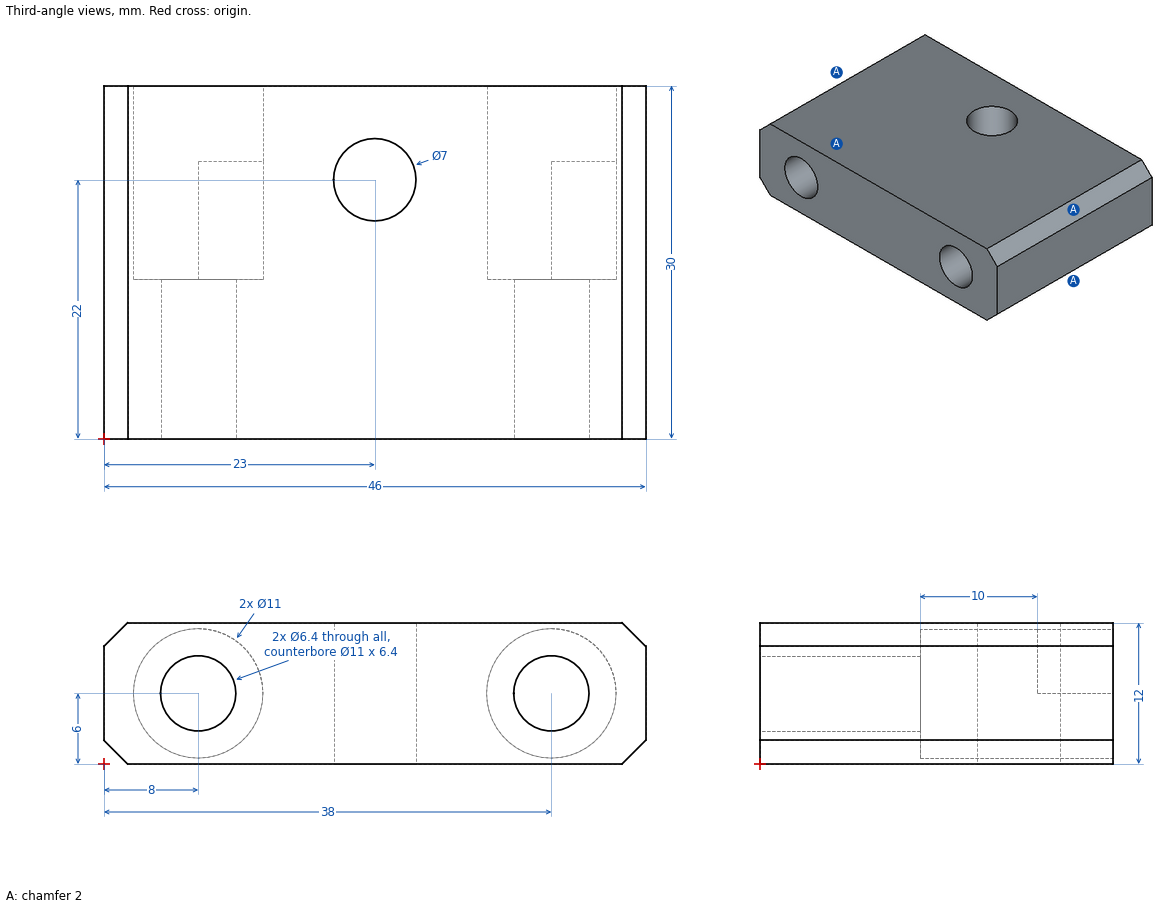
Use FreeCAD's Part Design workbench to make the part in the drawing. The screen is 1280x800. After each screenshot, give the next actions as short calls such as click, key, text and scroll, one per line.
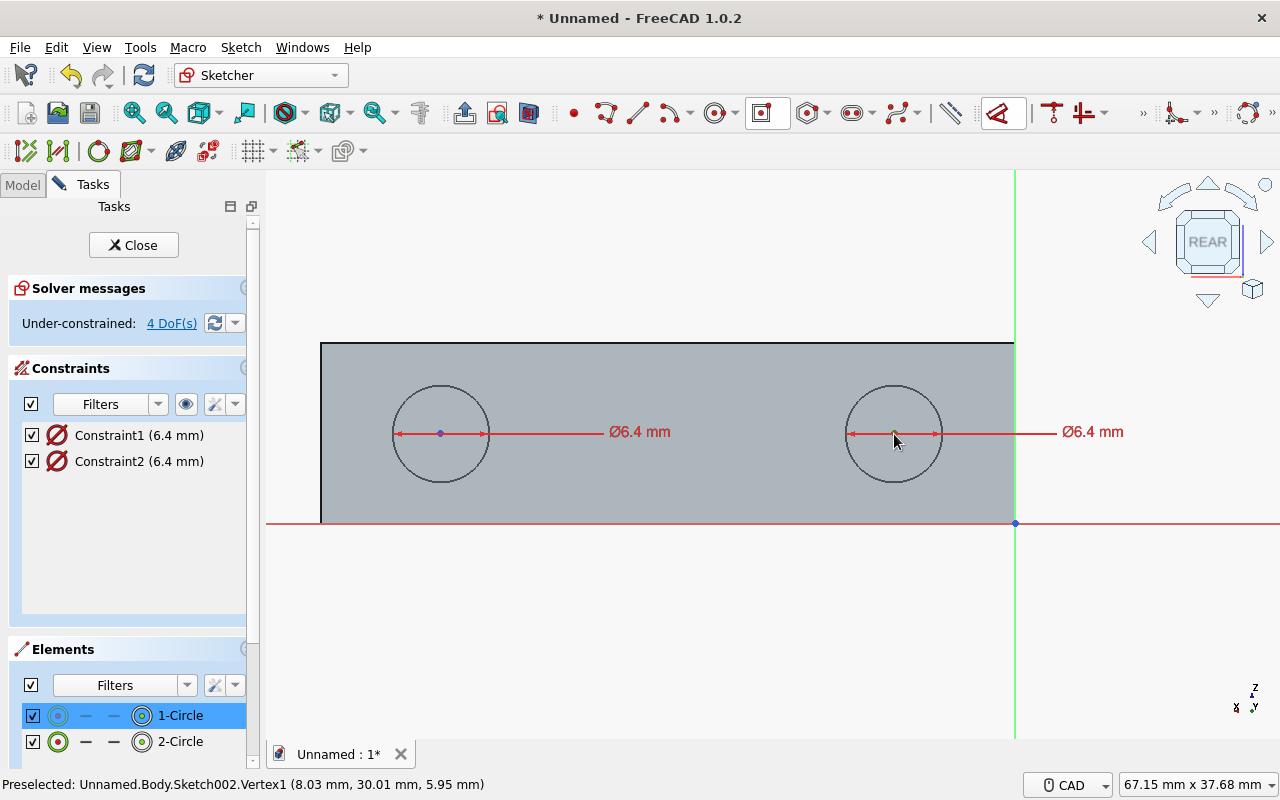
click(441, 434)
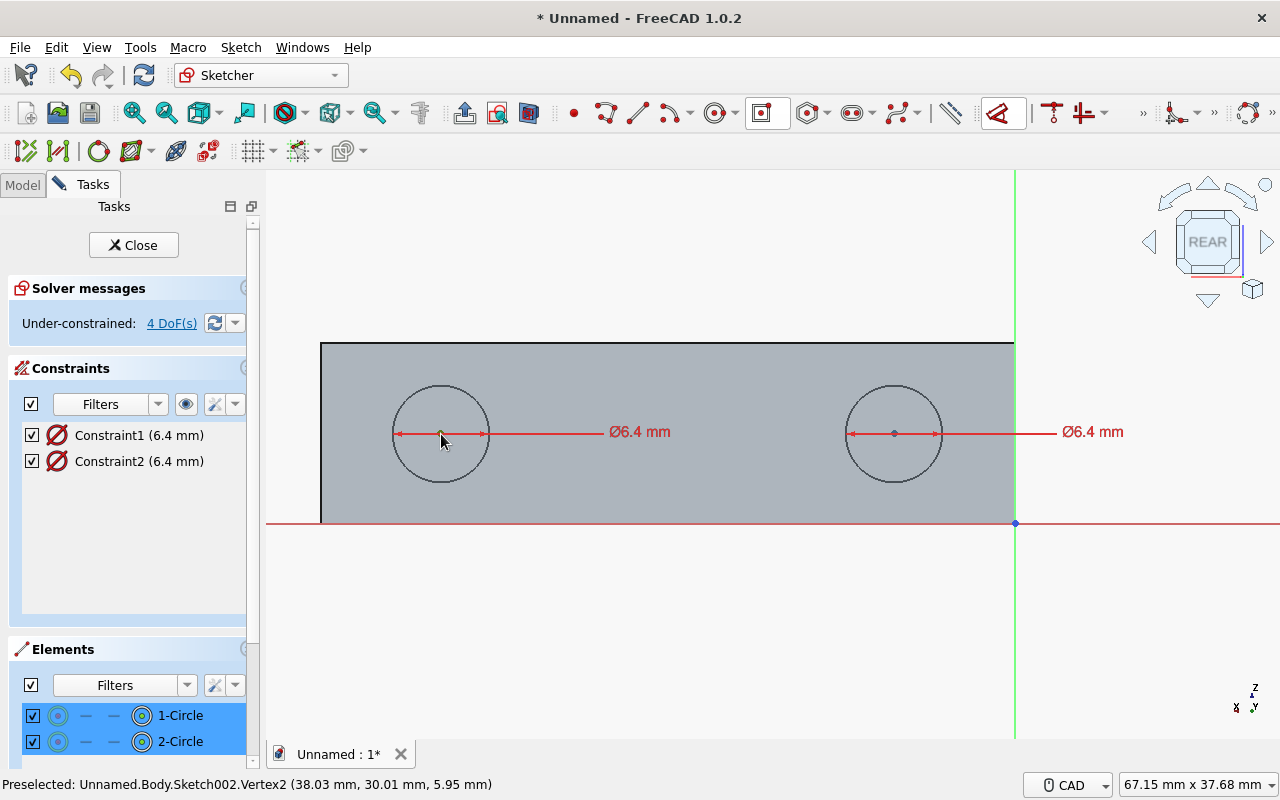
key(h)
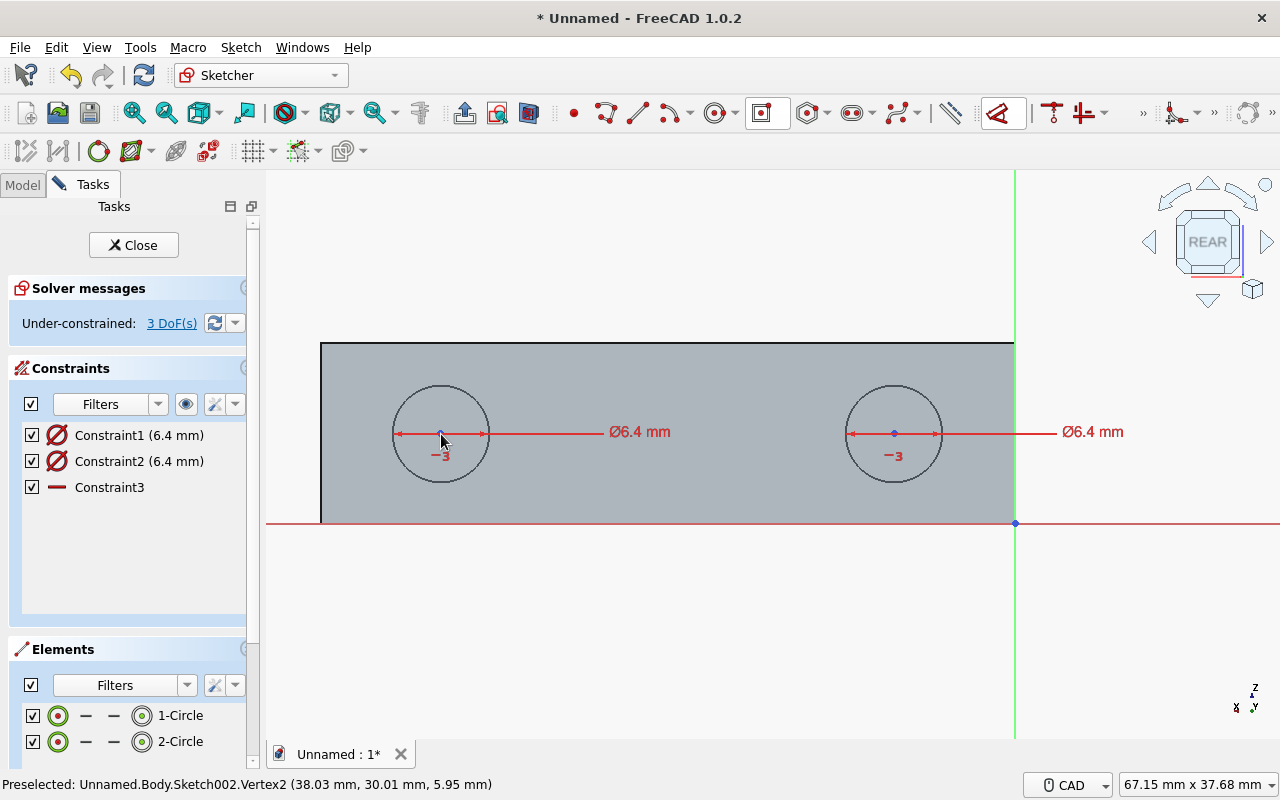
click(894, 434)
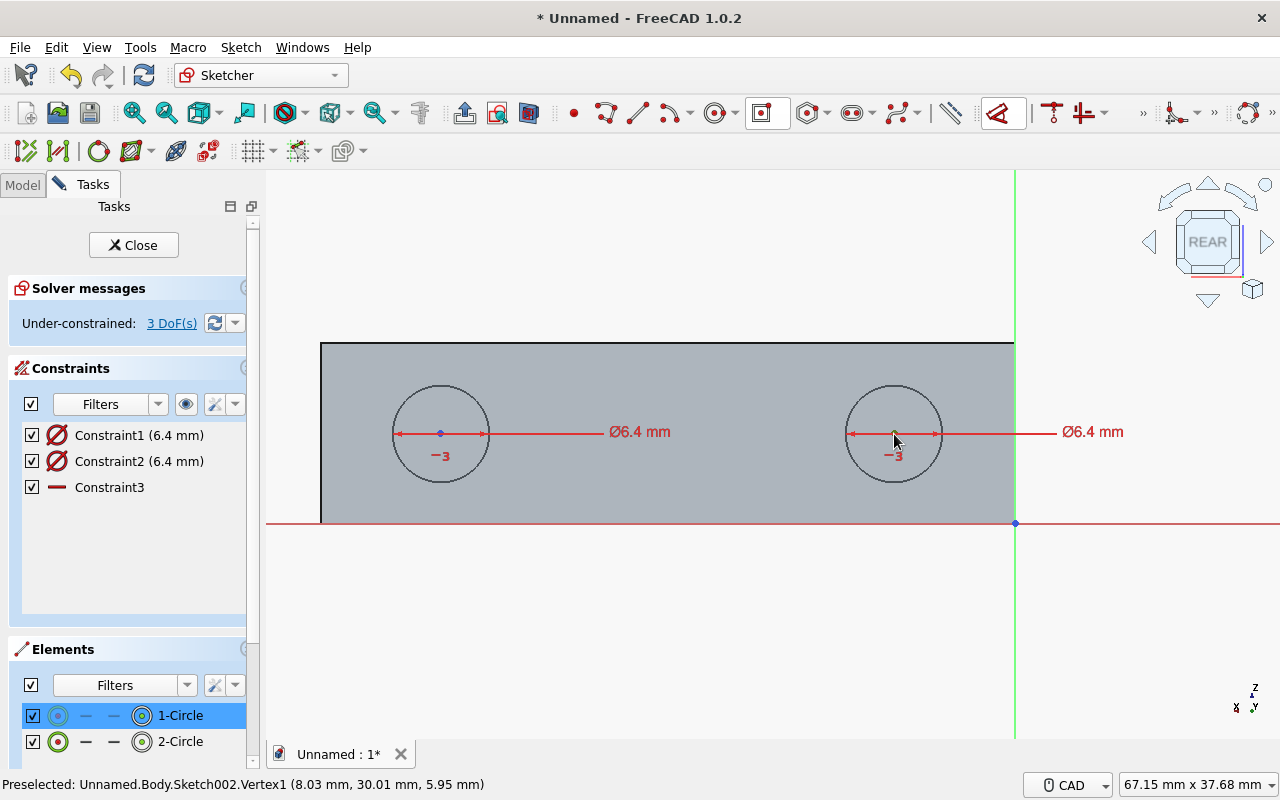
key(l)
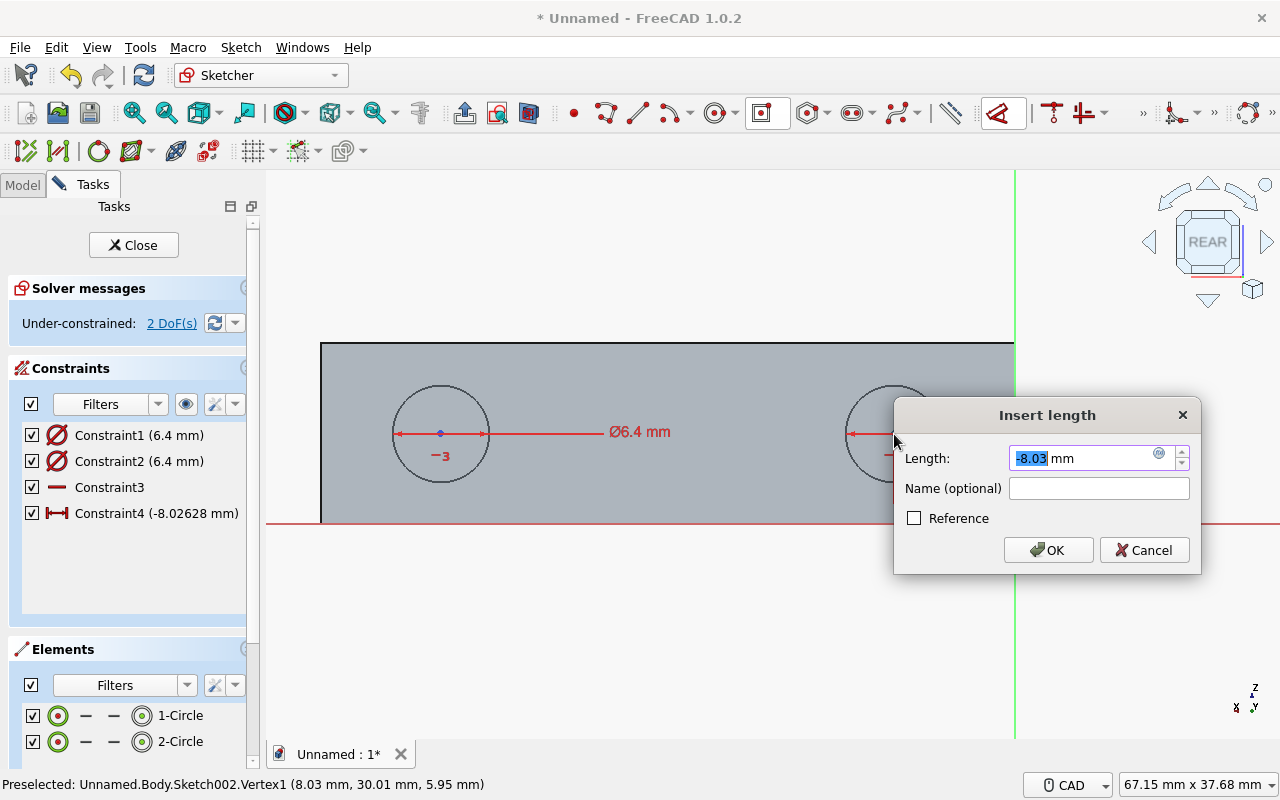
text(-8)
key(Return)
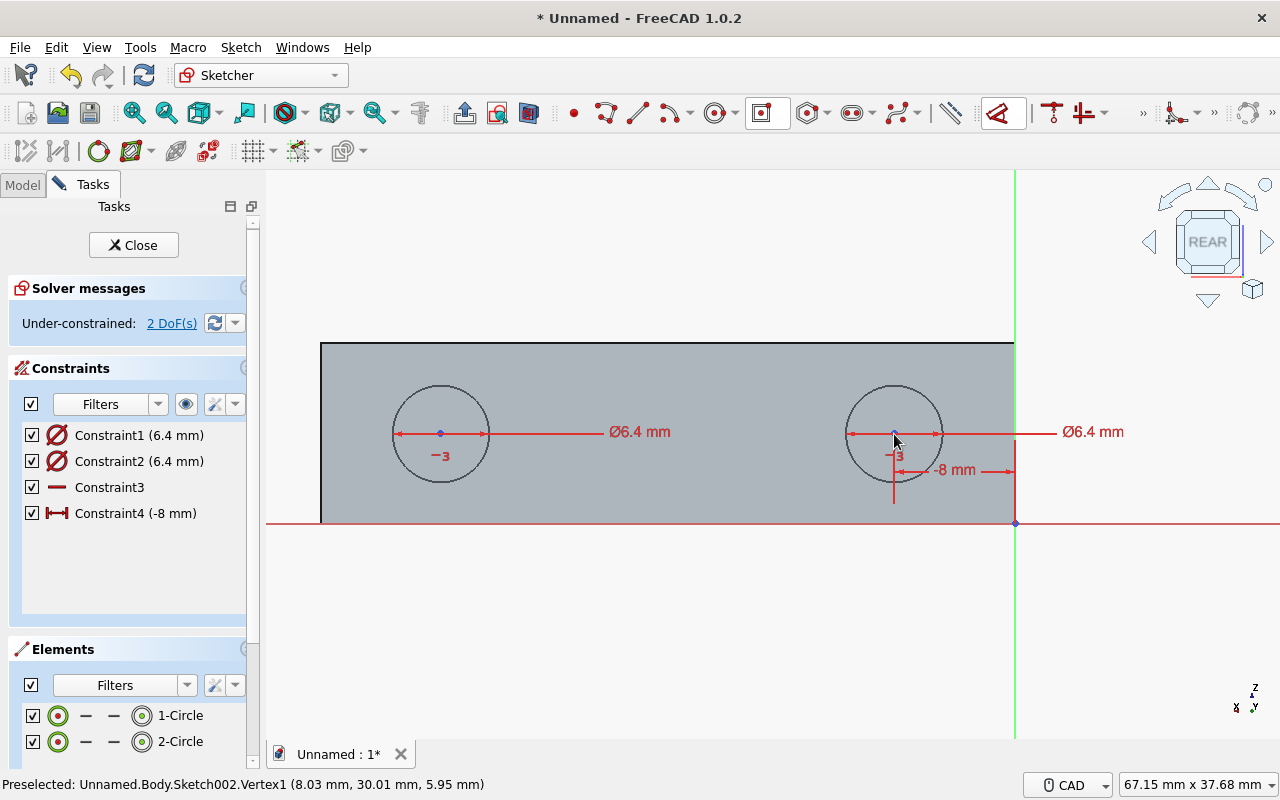
click(894, 434)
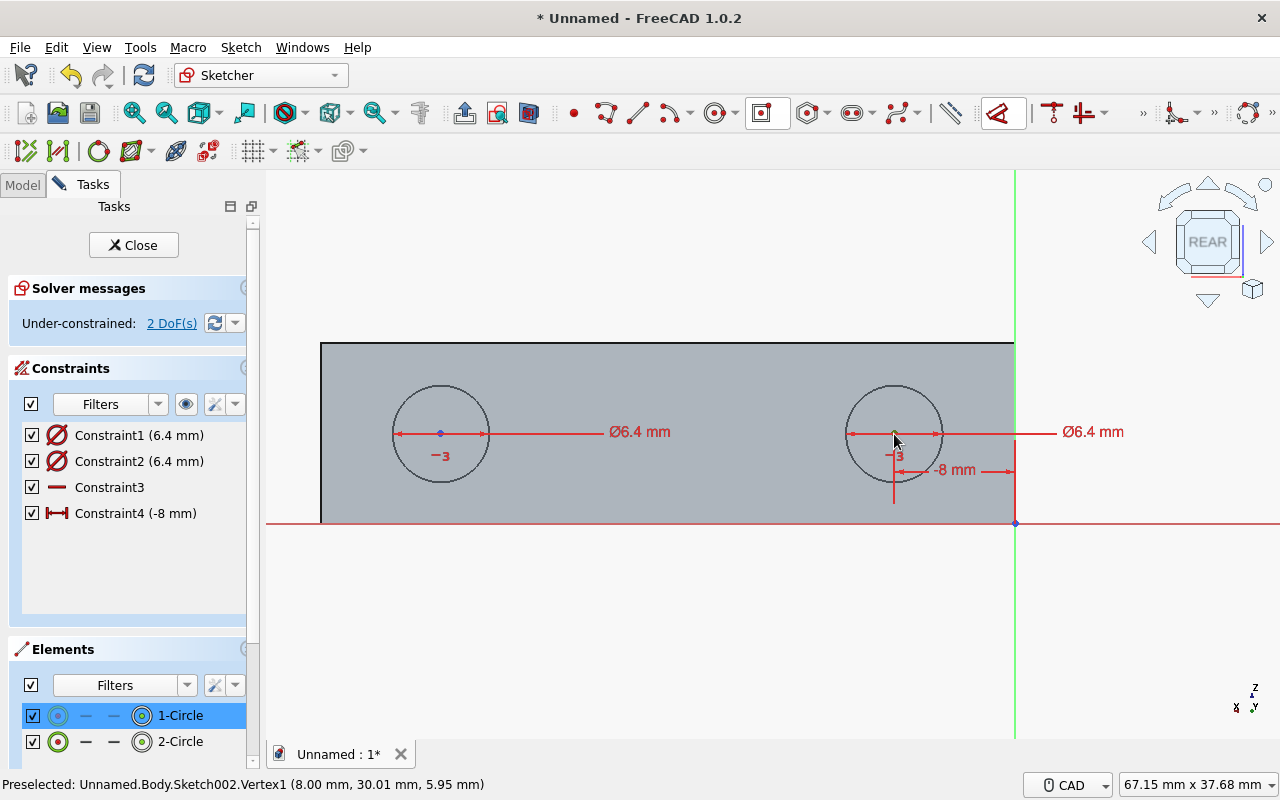
key(i)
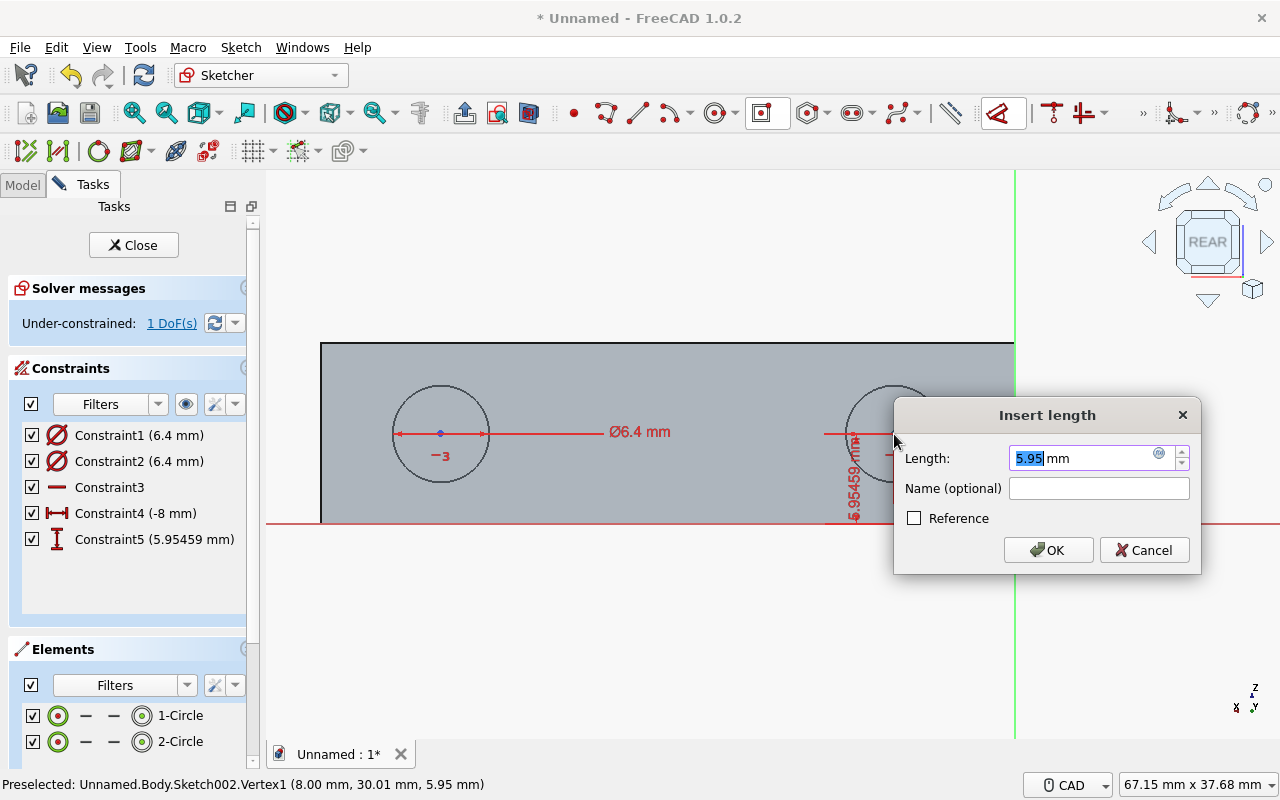
text(6)
key(Return)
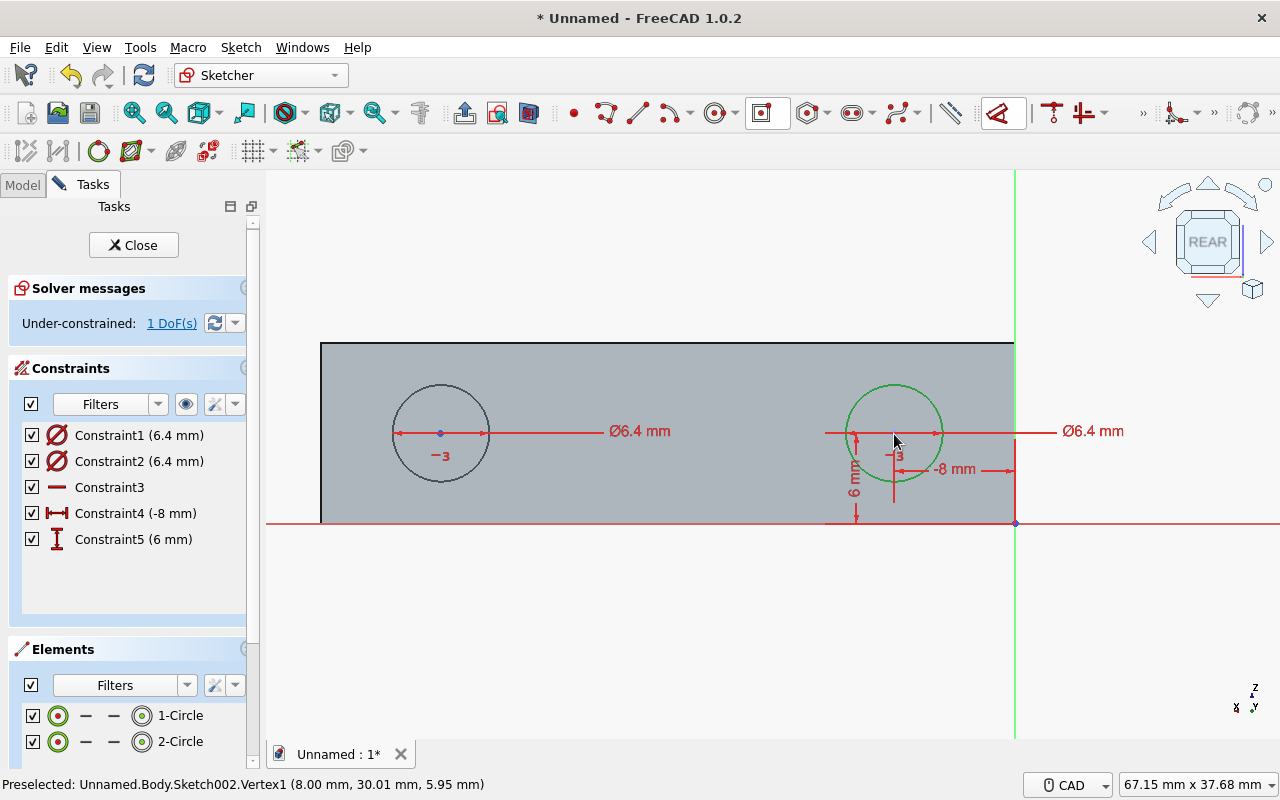
click(441, 433)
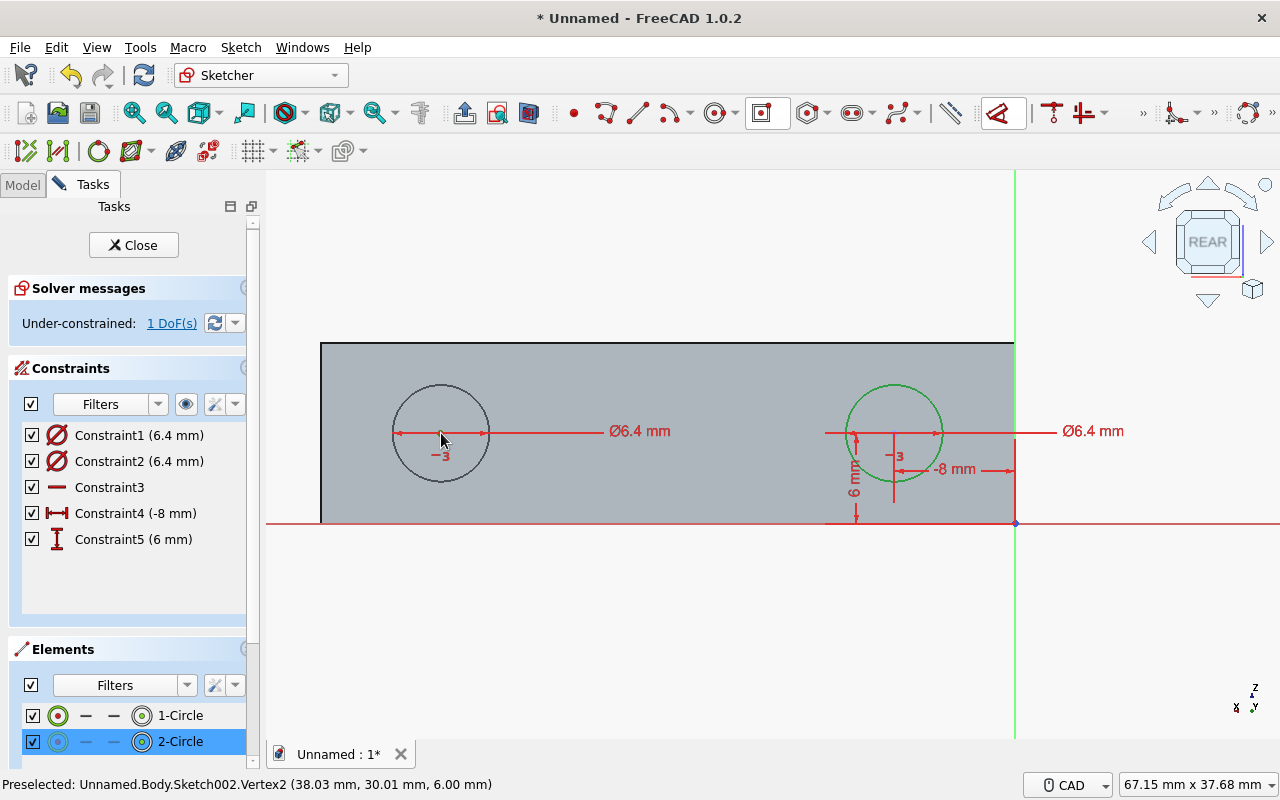
key(l)